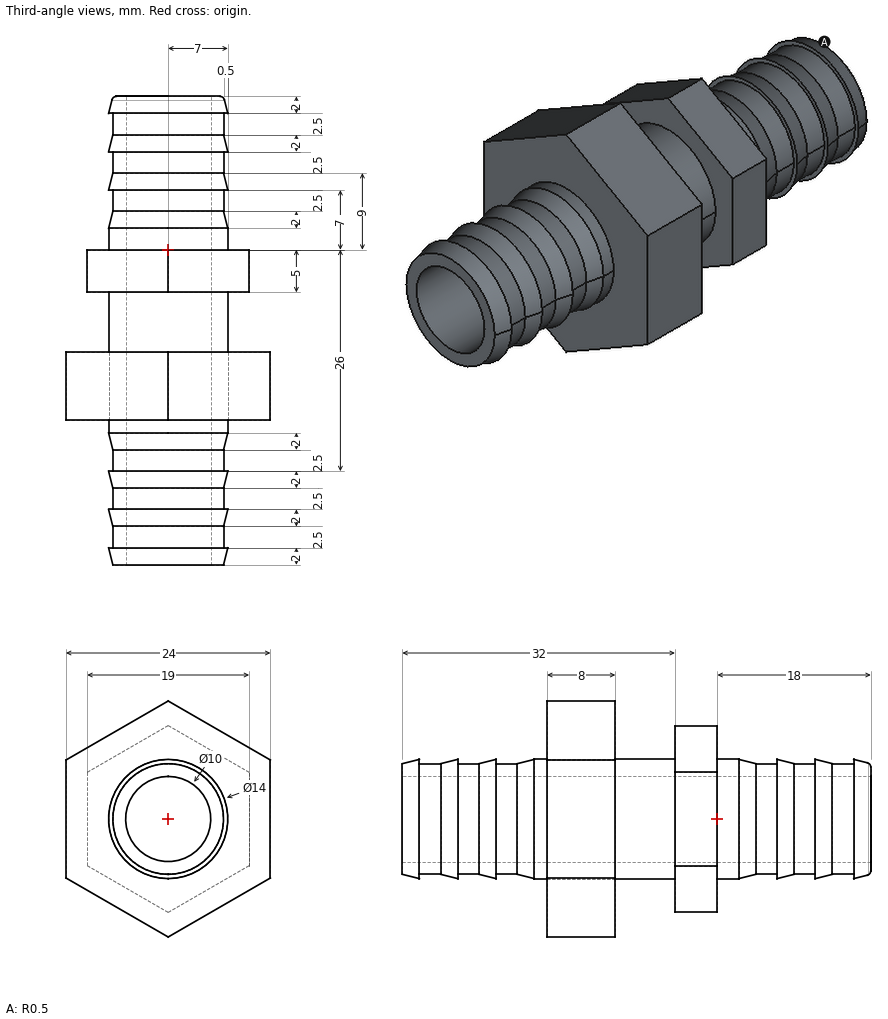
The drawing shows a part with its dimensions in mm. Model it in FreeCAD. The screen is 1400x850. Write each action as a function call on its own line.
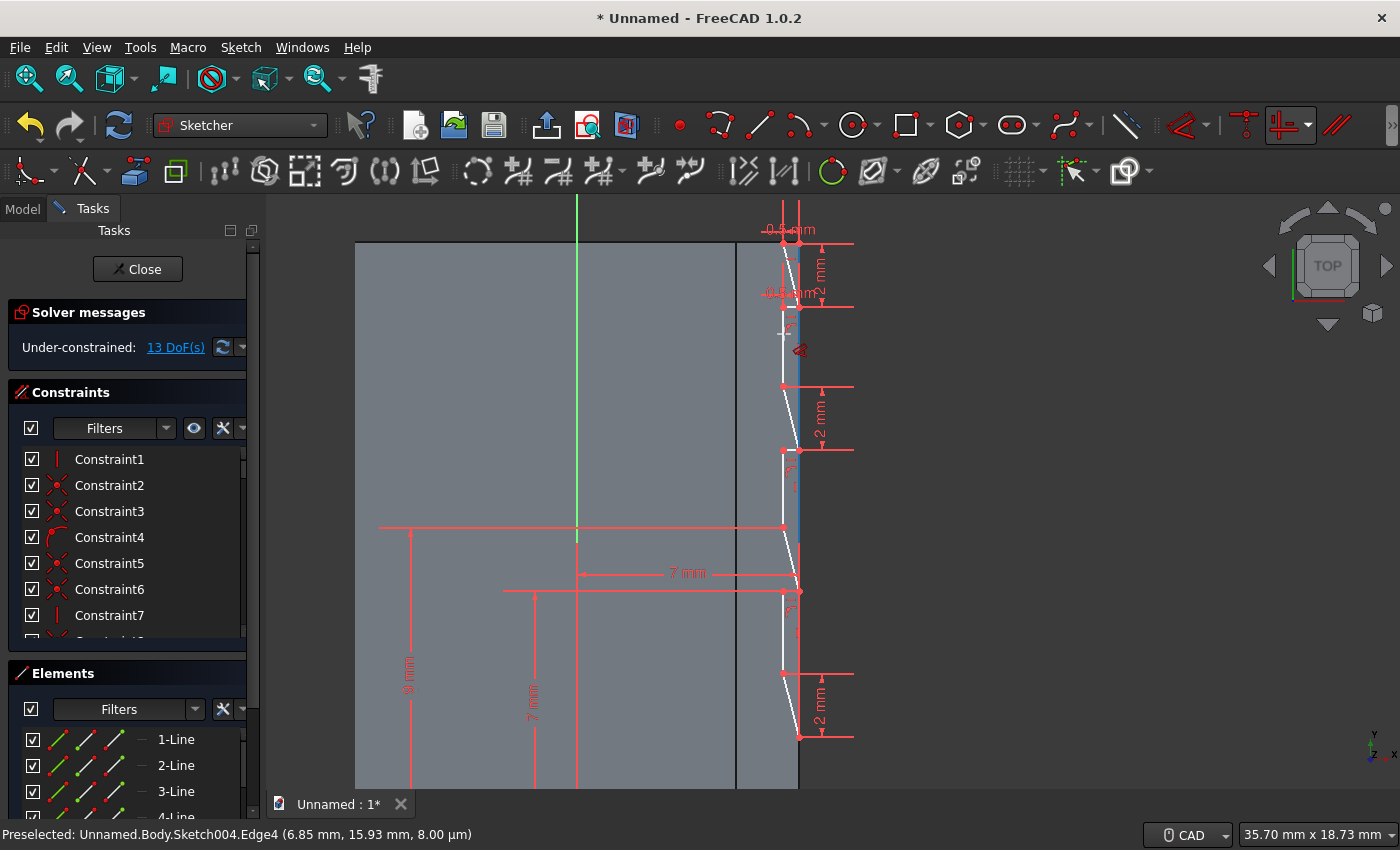
click(783, 331)
click(817, 347)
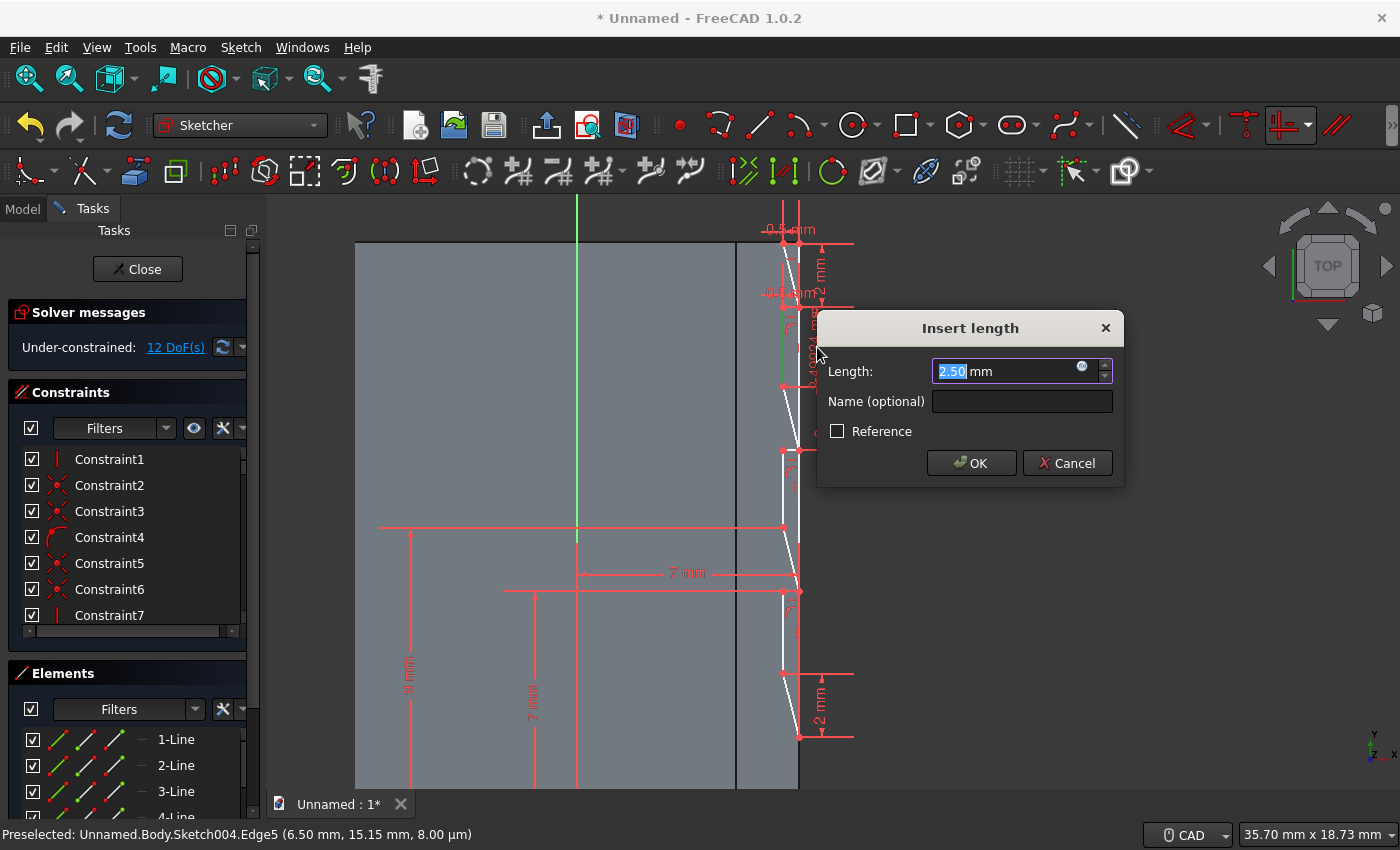
text(2.5)
key(Return)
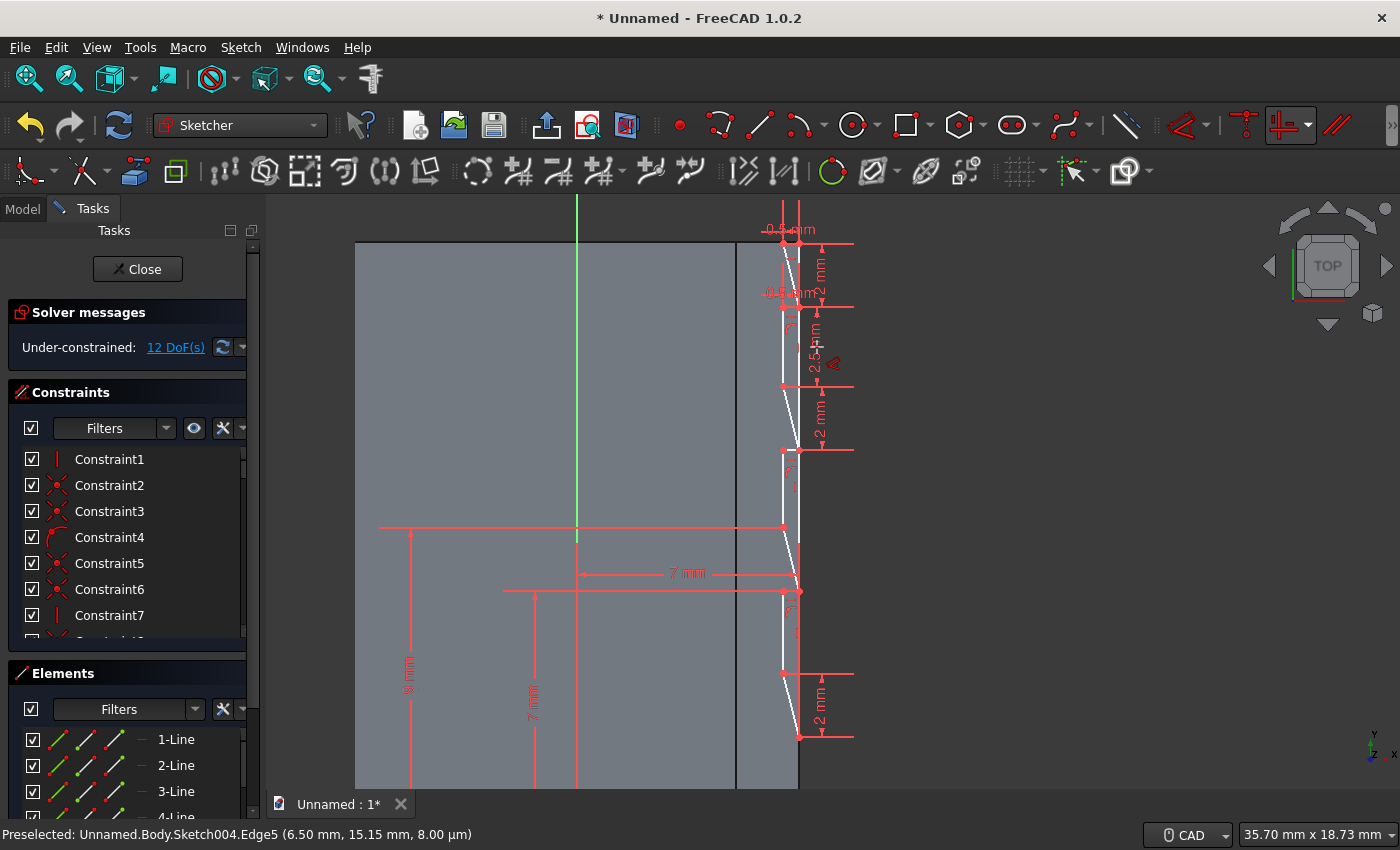
scroll(791, 450, up, 5)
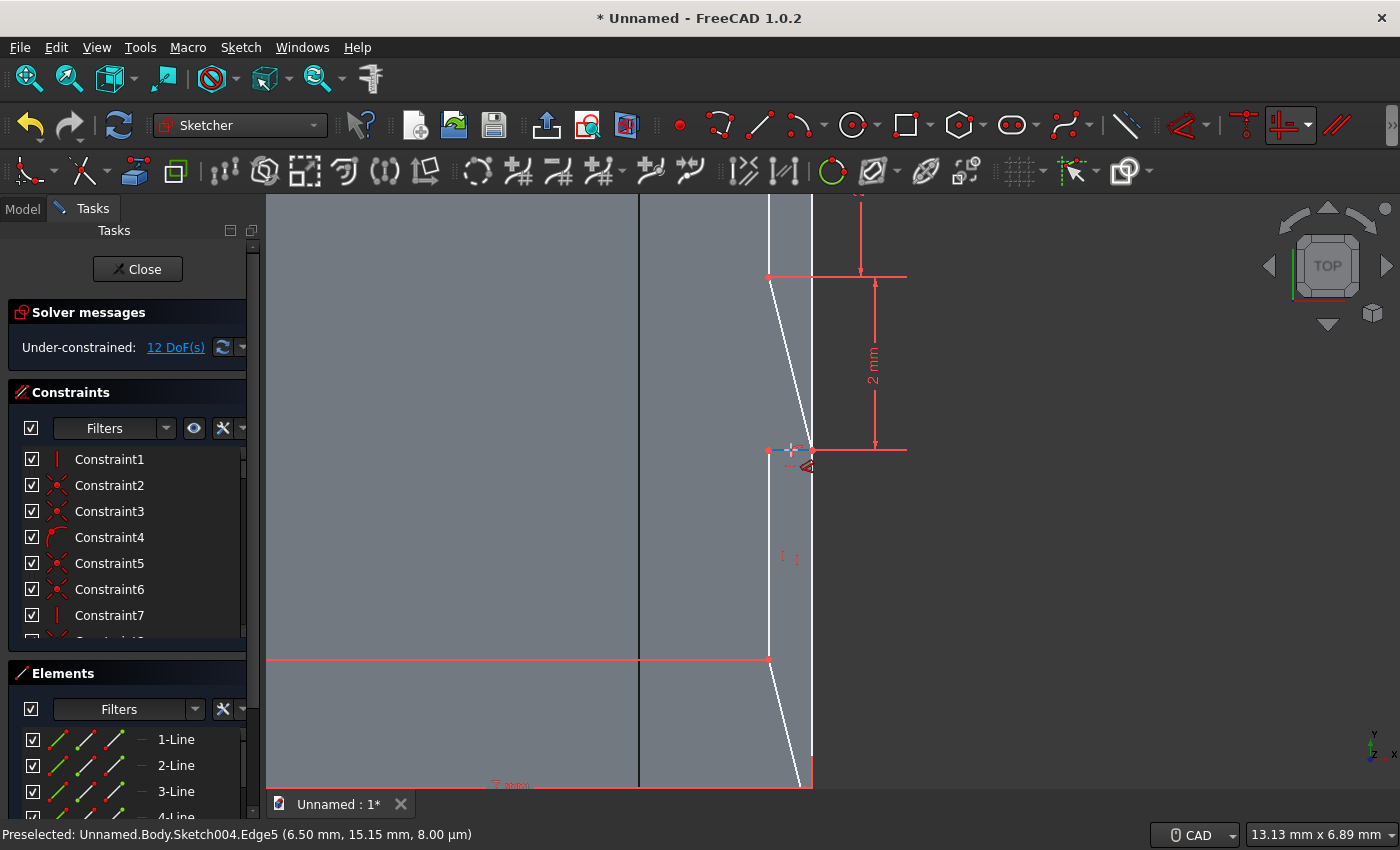
click(790, 450)
click(780, 416)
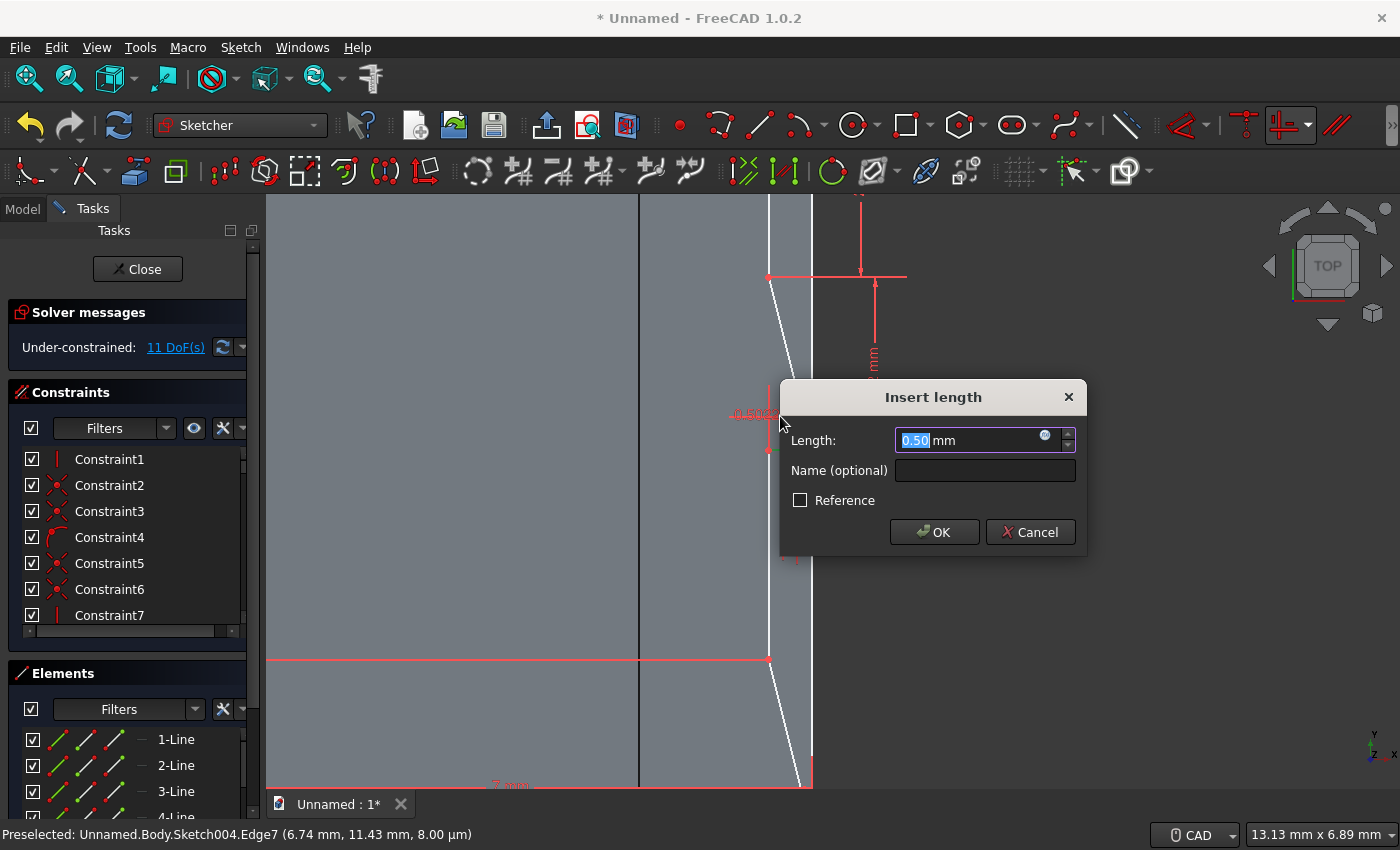
text(0.5)
key(Return)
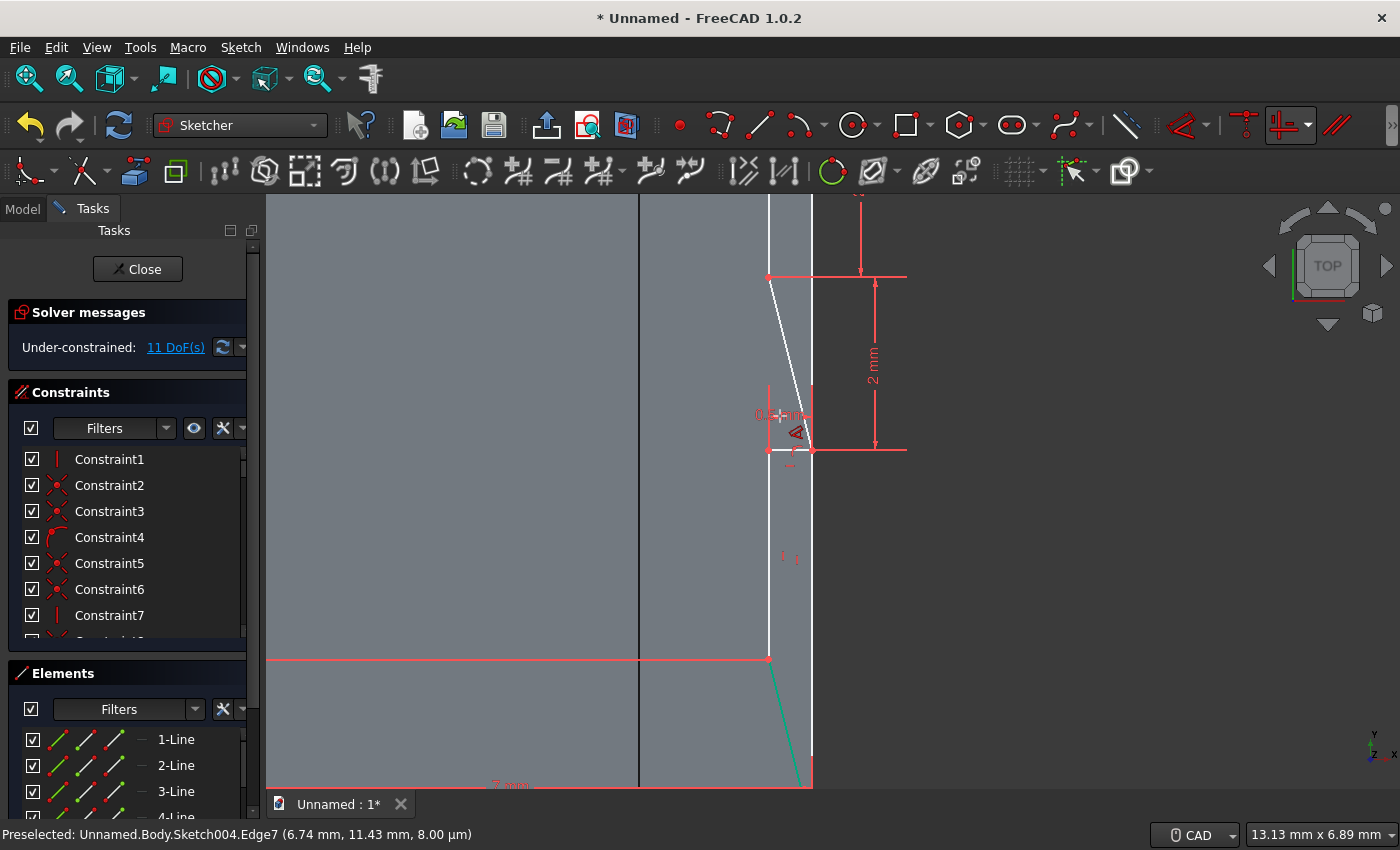
scroll(785, 350, down, 13)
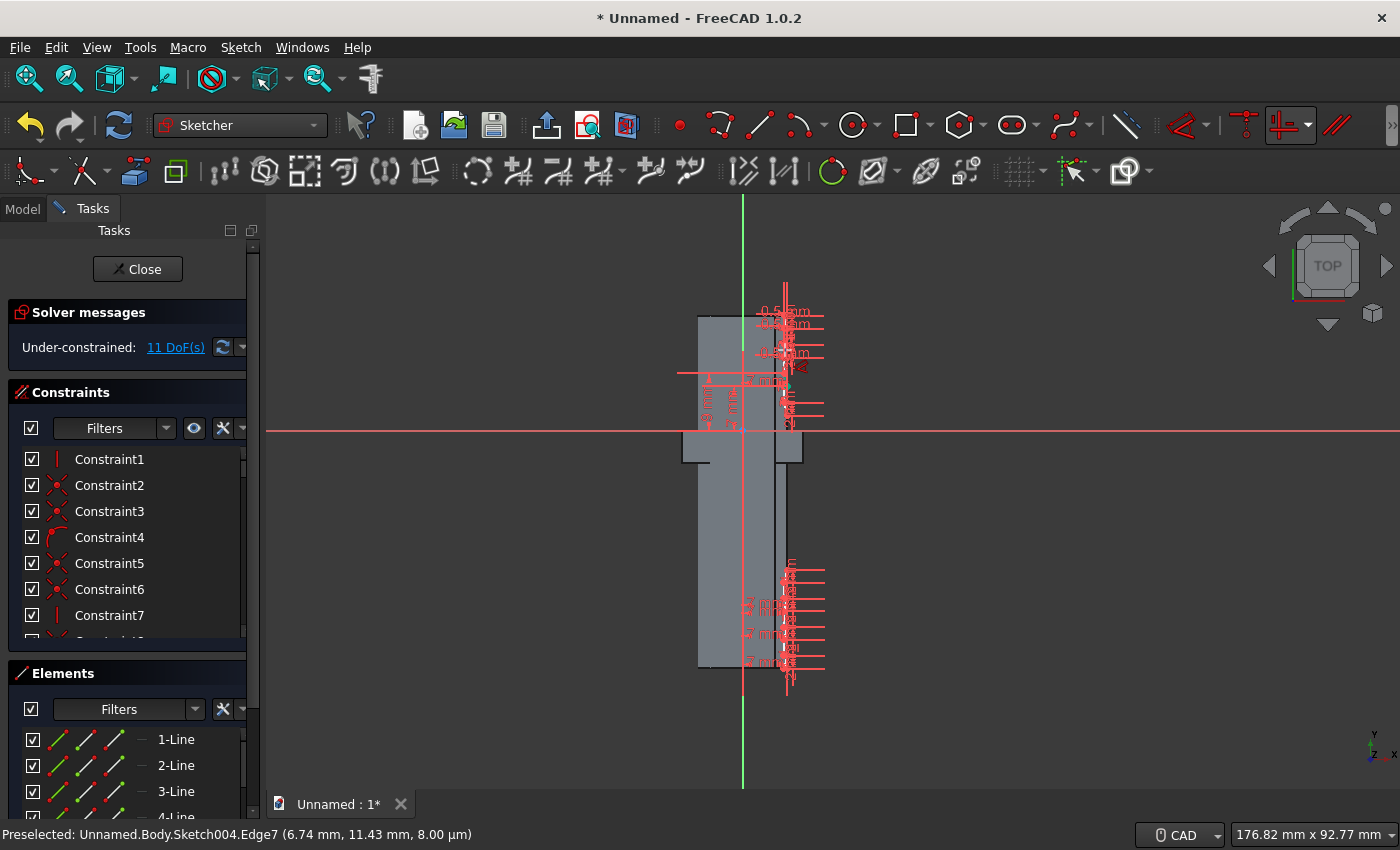
scroll(784, 362, up, 8)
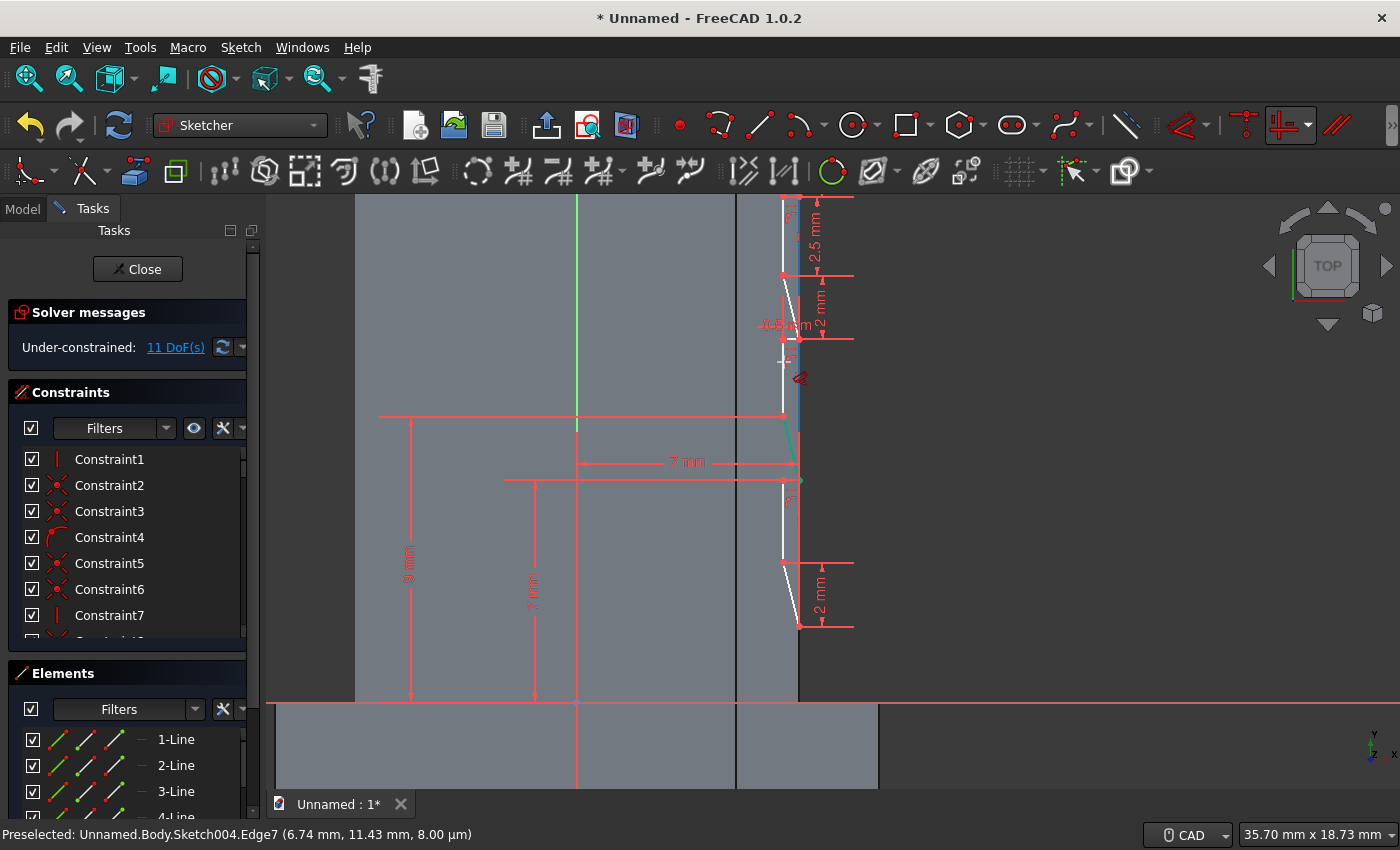
click(783, 363)
click(817, 378)